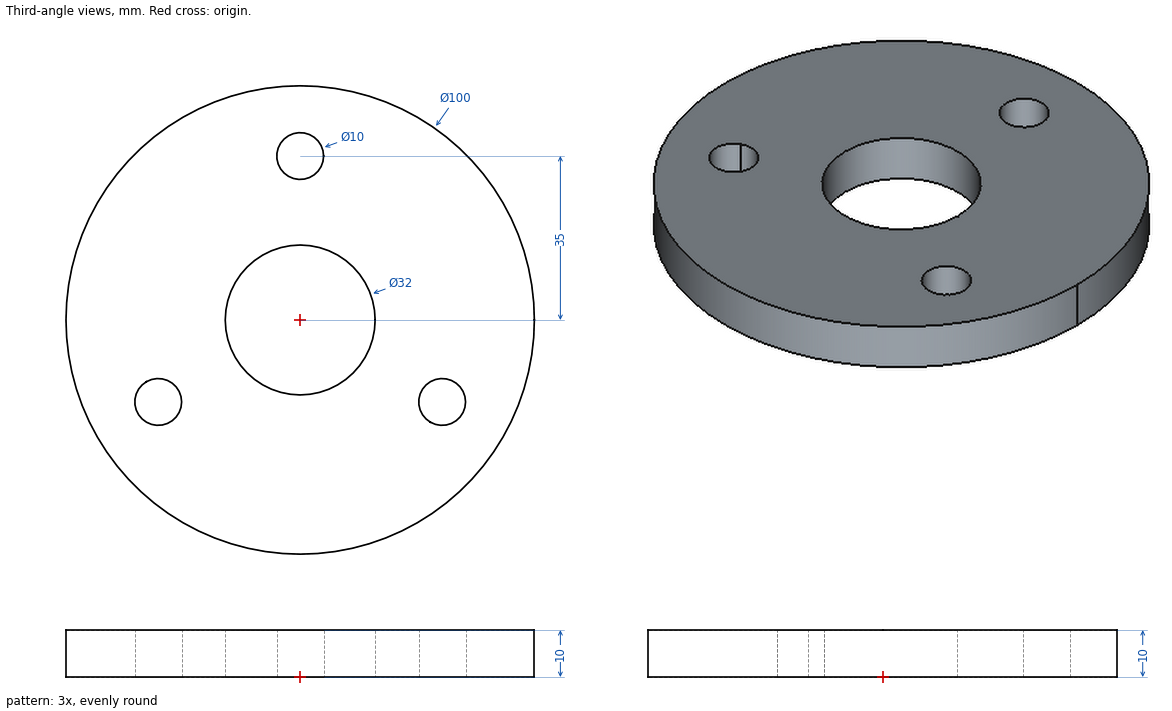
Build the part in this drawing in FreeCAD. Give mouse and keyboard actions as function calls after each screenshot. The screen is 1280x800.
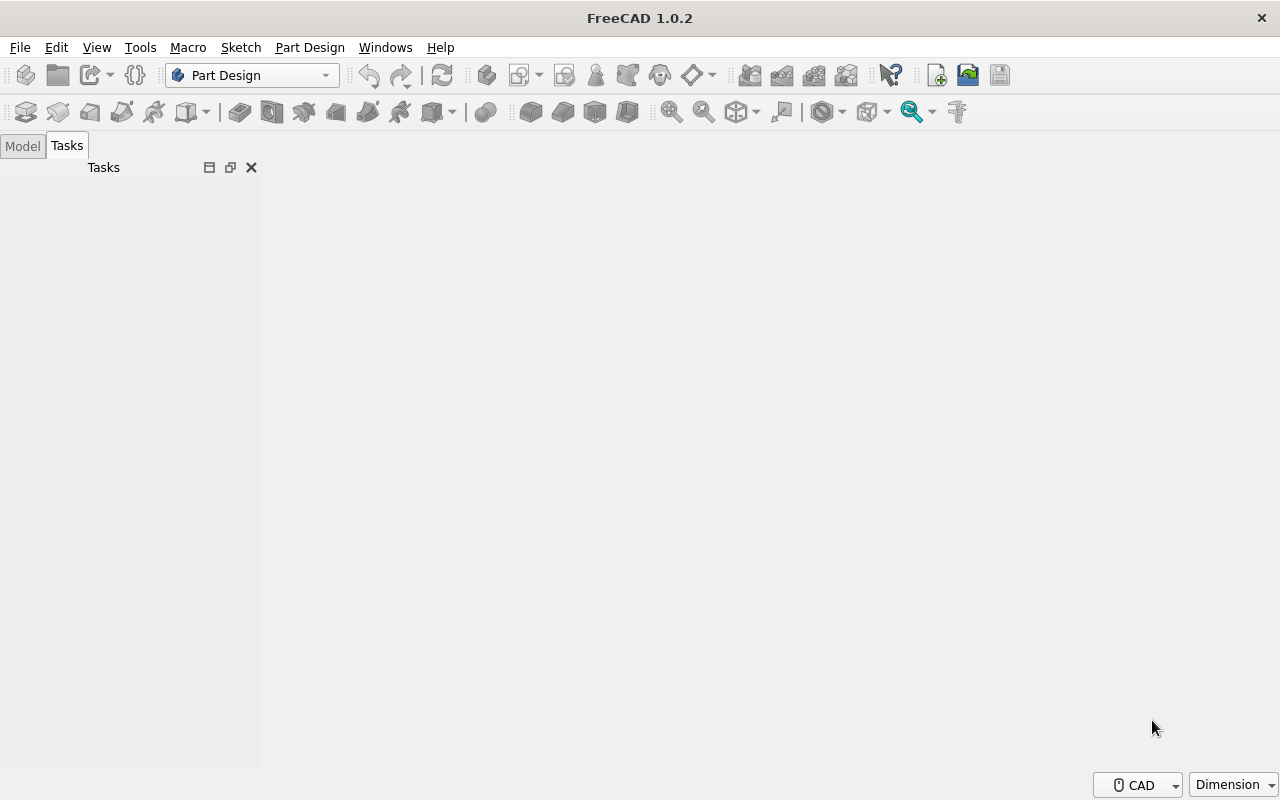
click(936, 76)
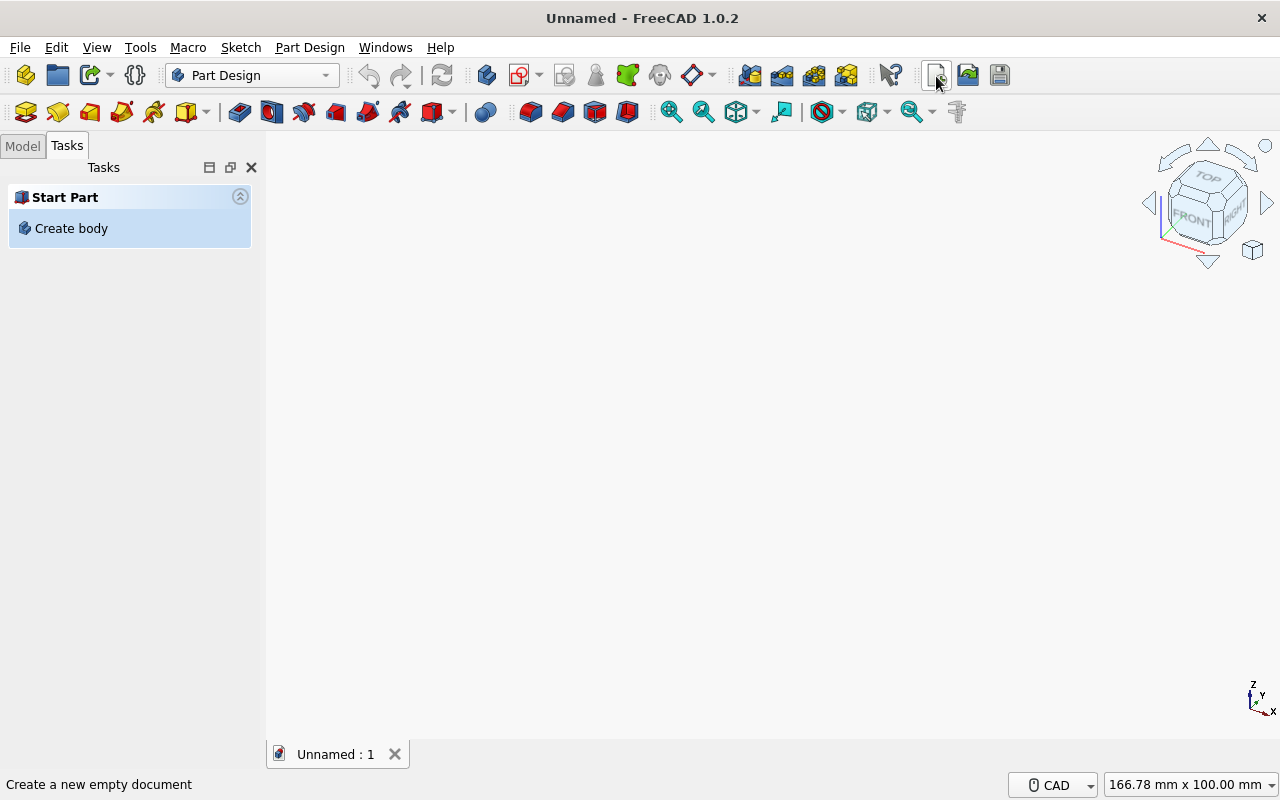
click(520, 76)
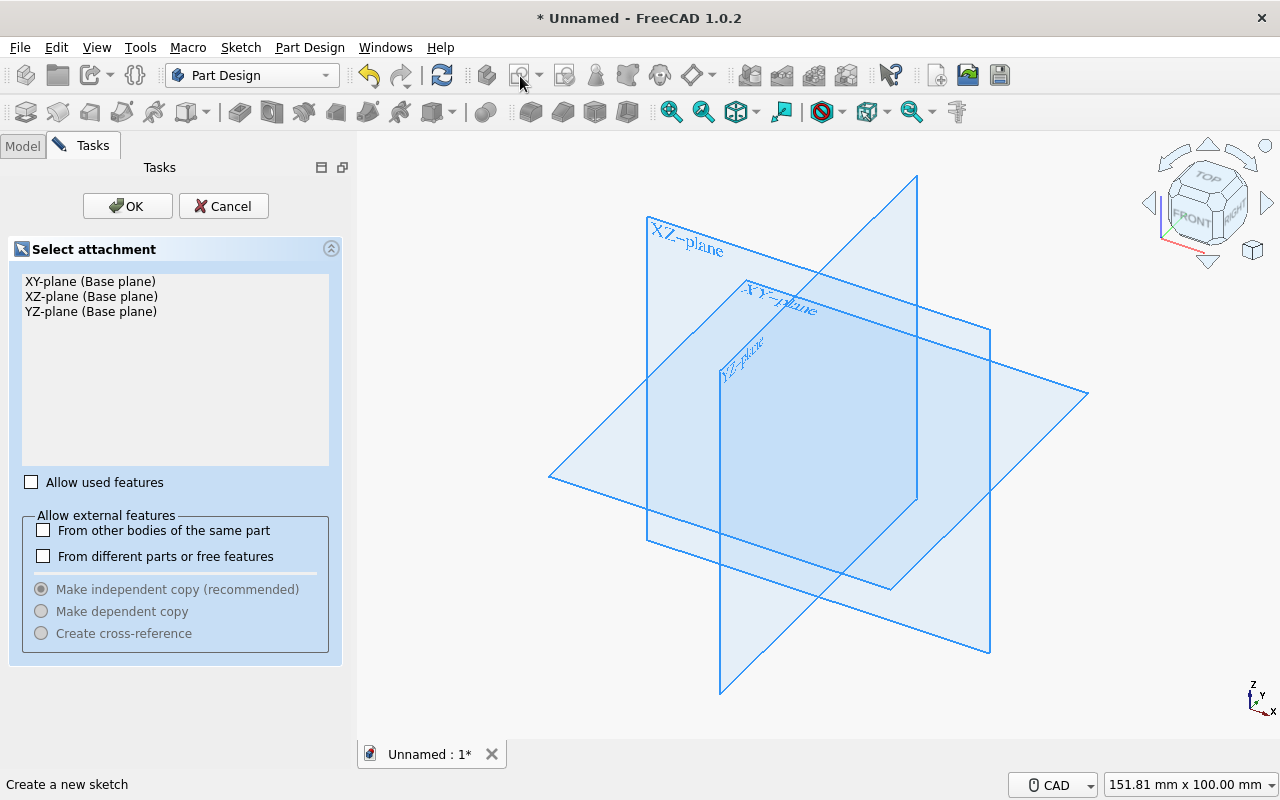
click(82, 282)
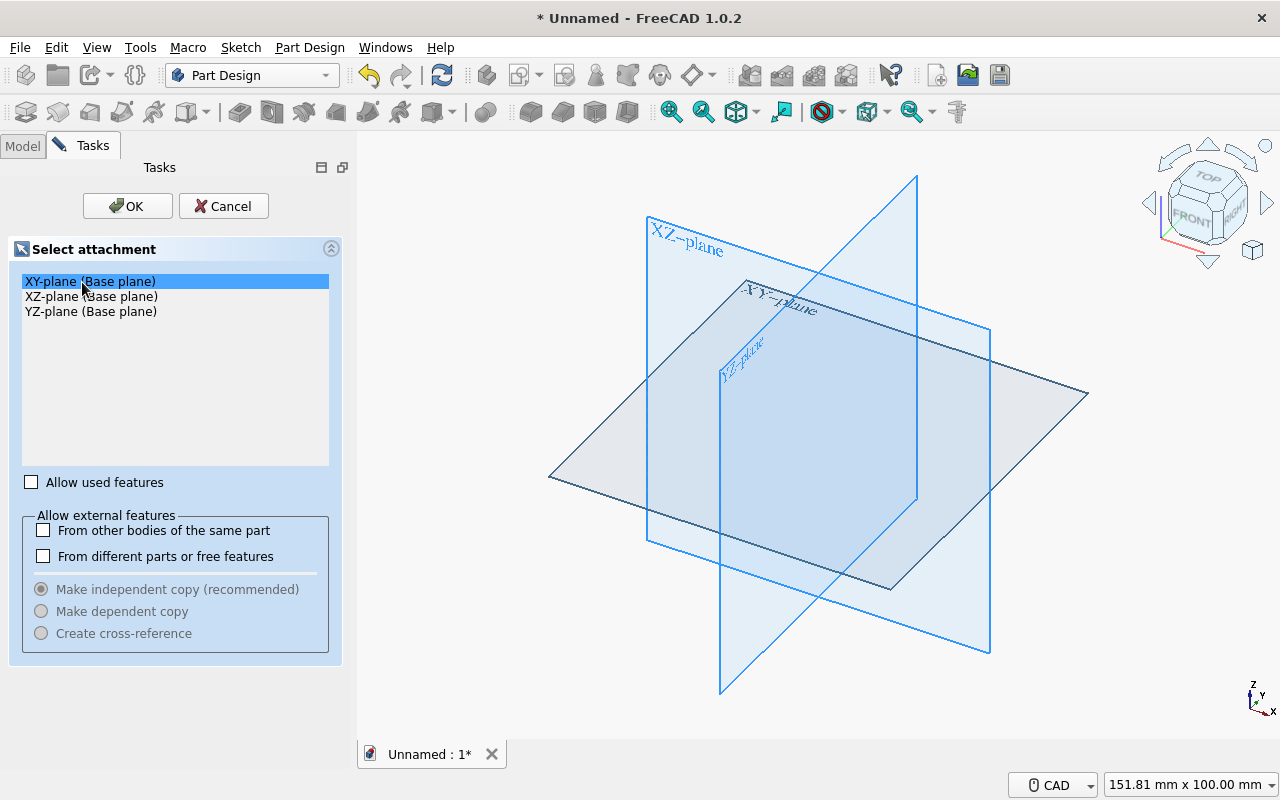
click(128, 206)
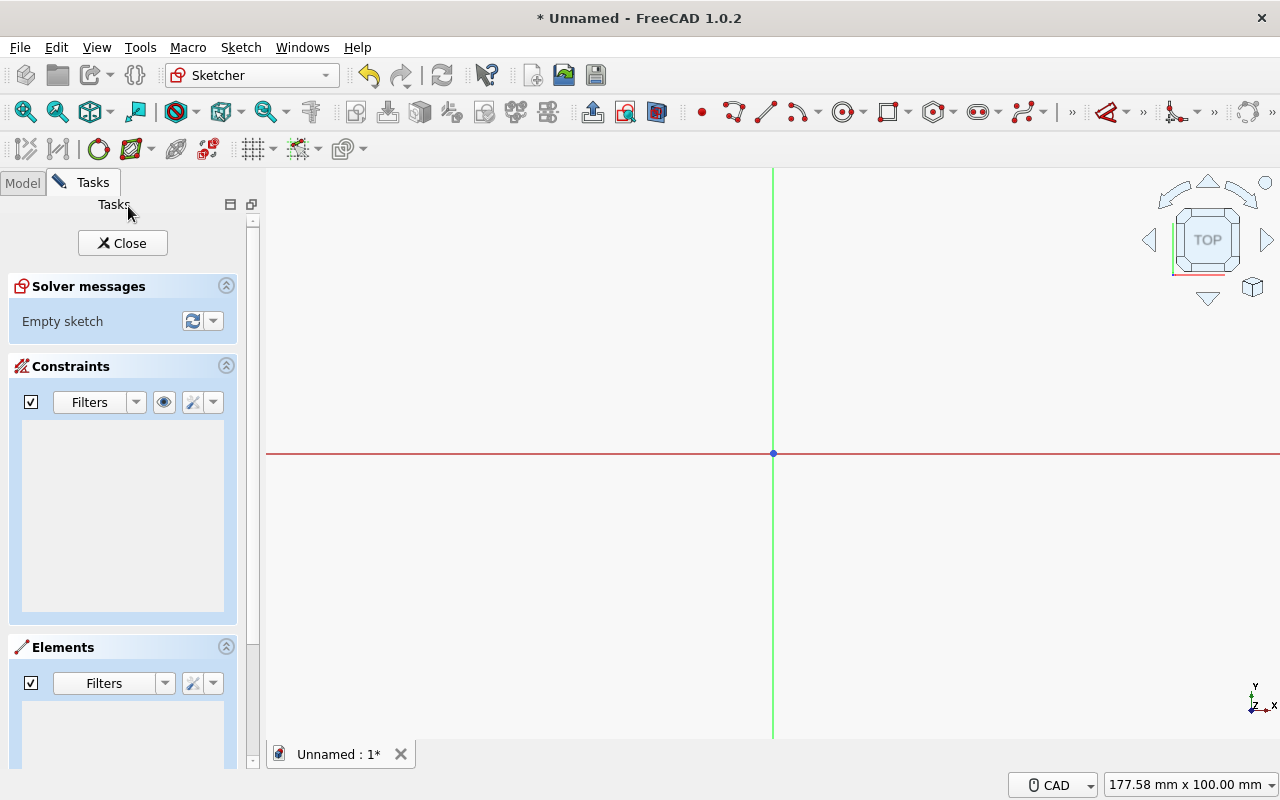
scroll(565, 453, down, 2)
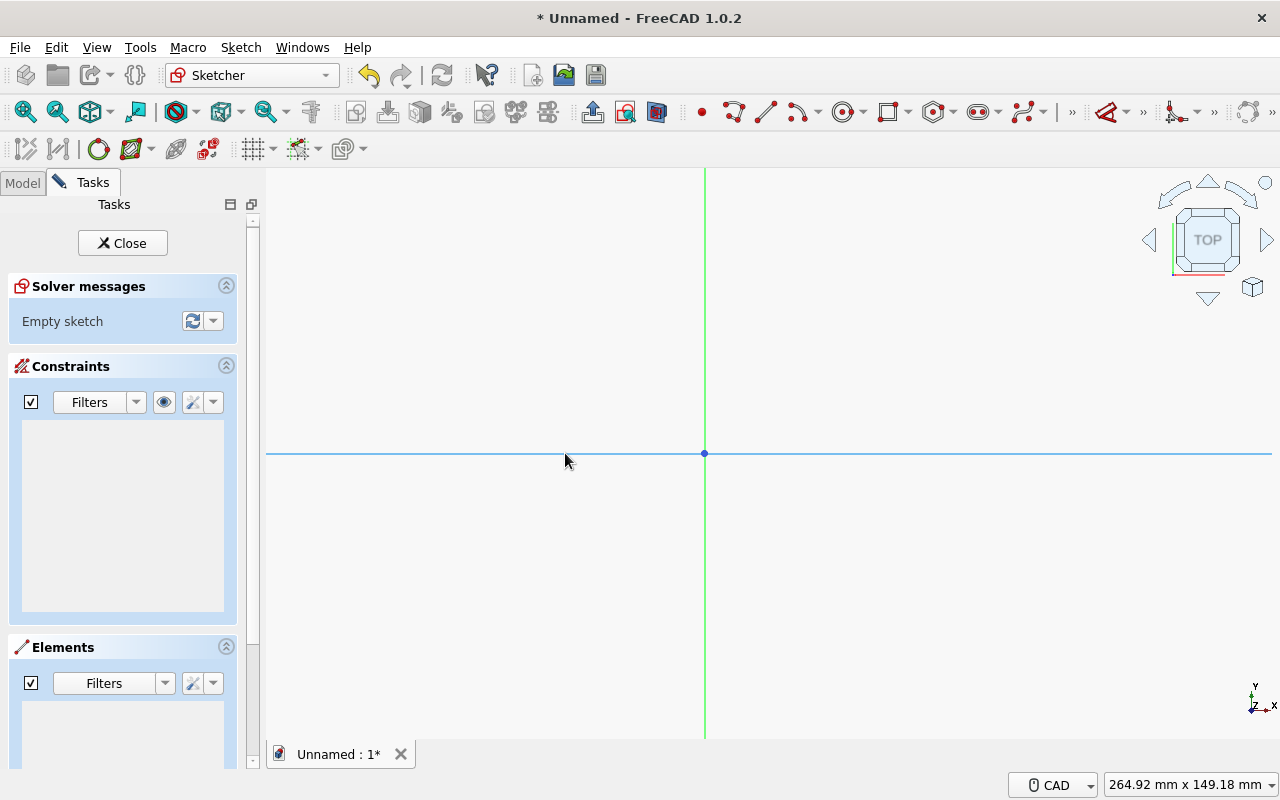
click(844, 112)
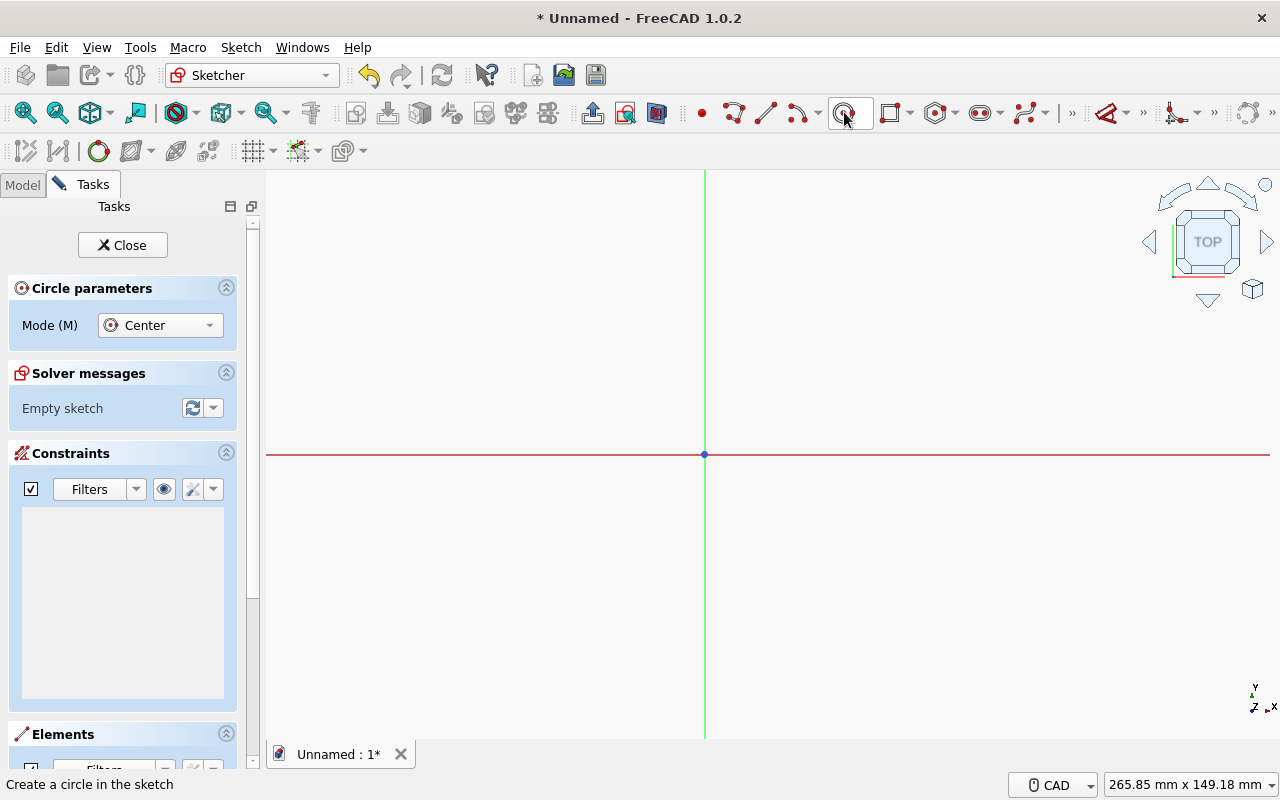
click(705, 454)
move(840, 320)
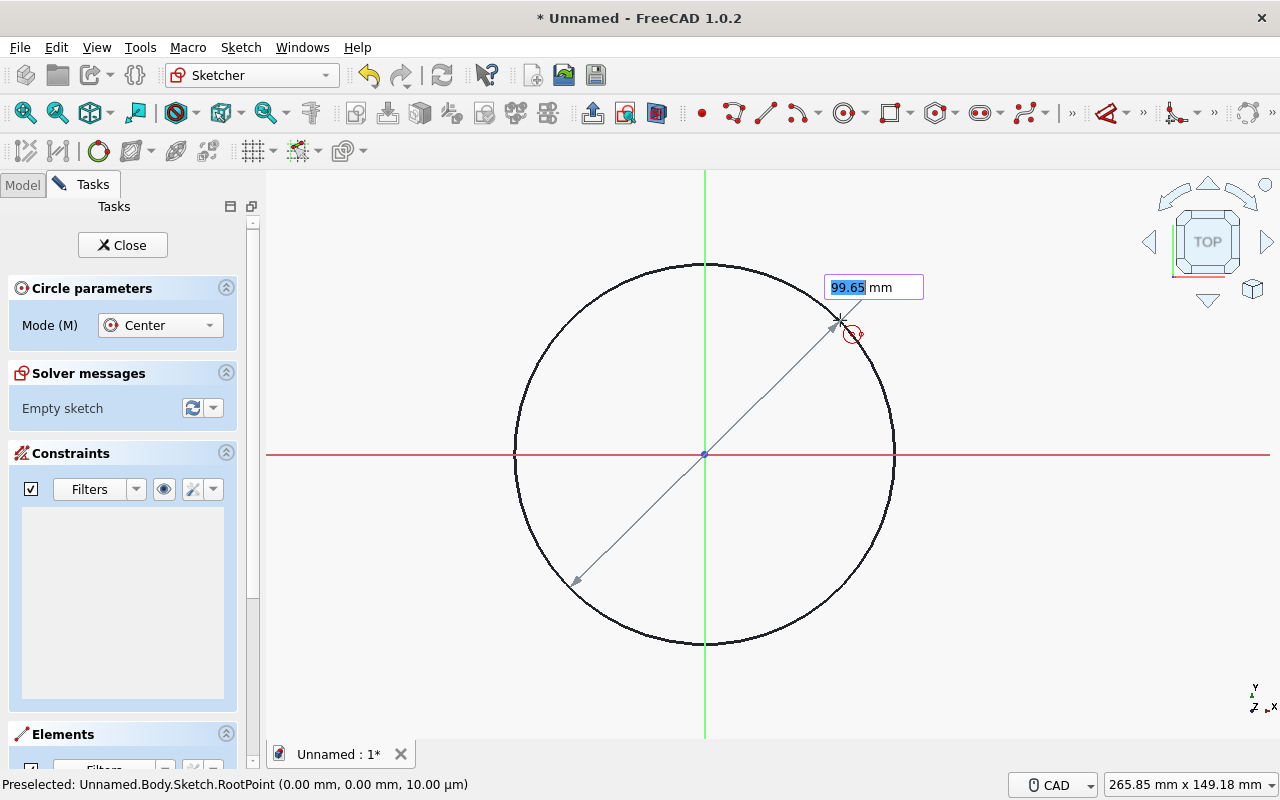
text(100)
key(Return)
key(Escape)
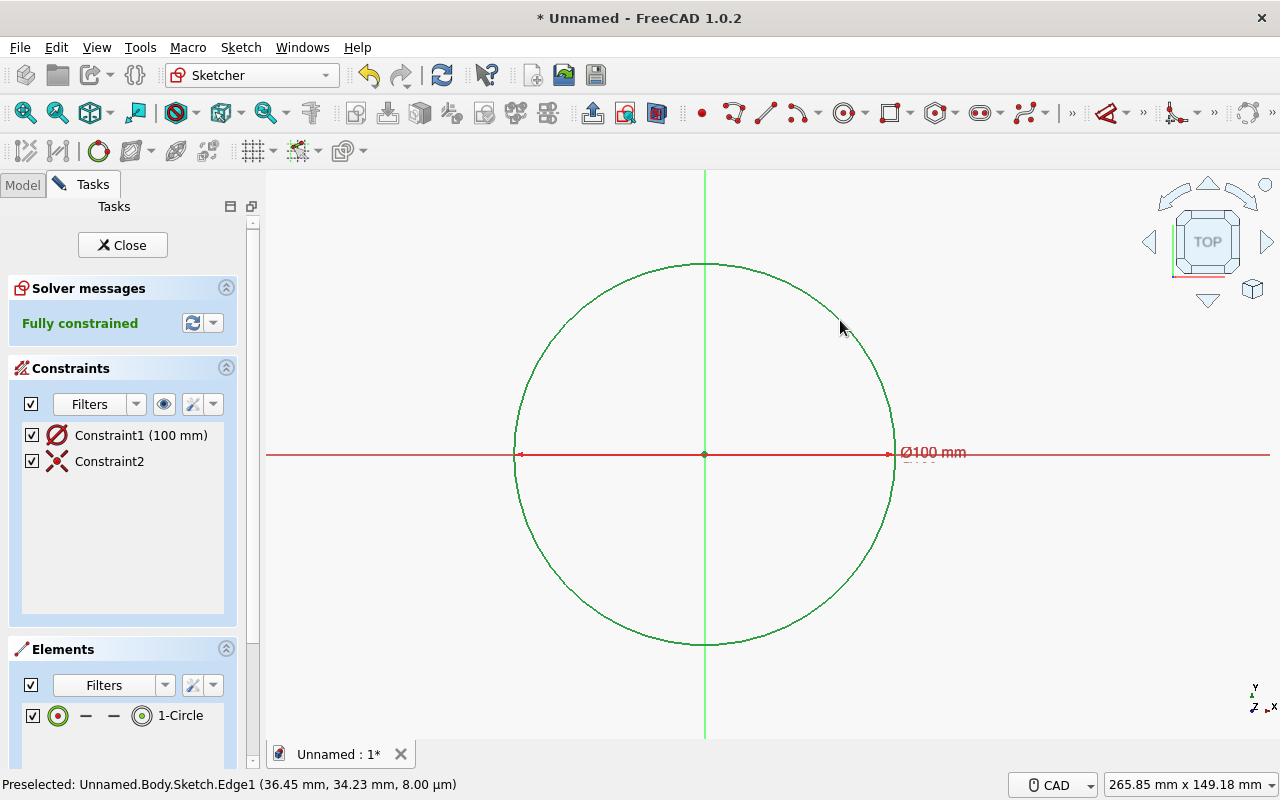
click(123, 245)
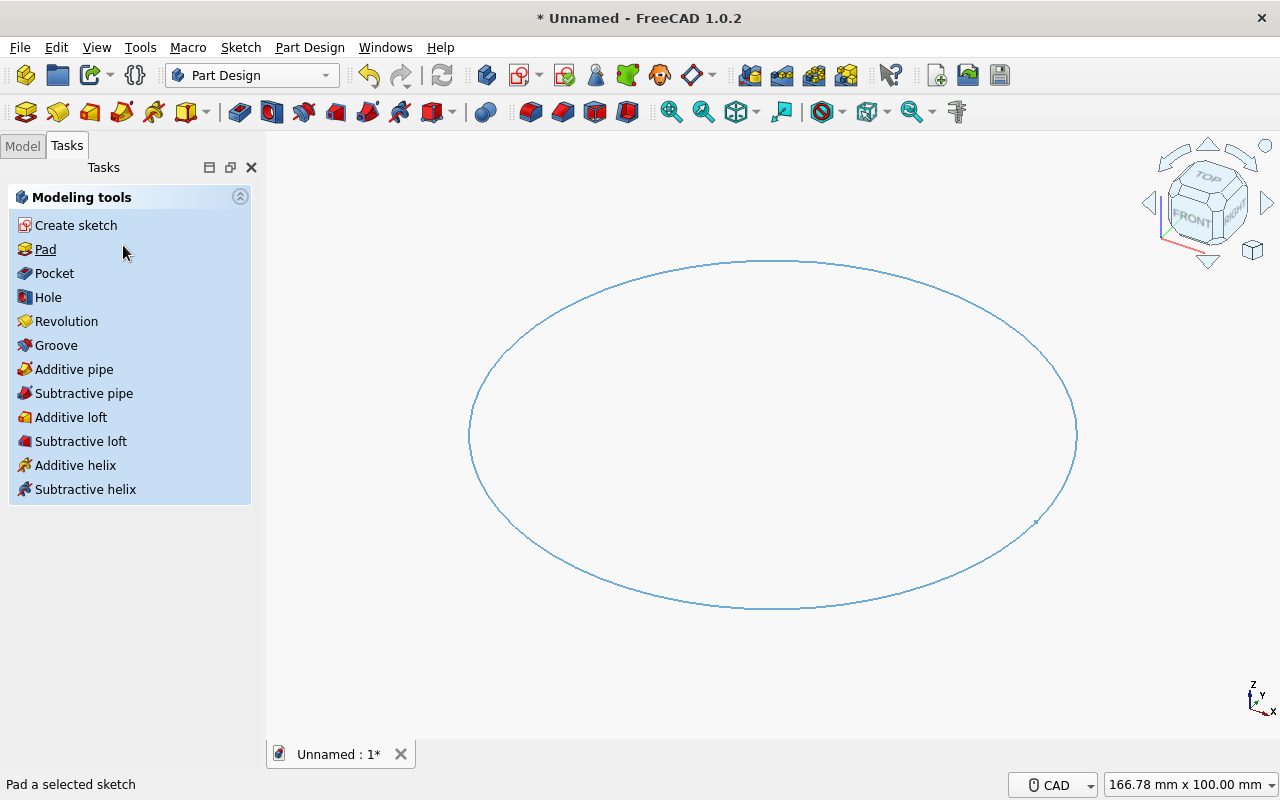
click(26, 112)